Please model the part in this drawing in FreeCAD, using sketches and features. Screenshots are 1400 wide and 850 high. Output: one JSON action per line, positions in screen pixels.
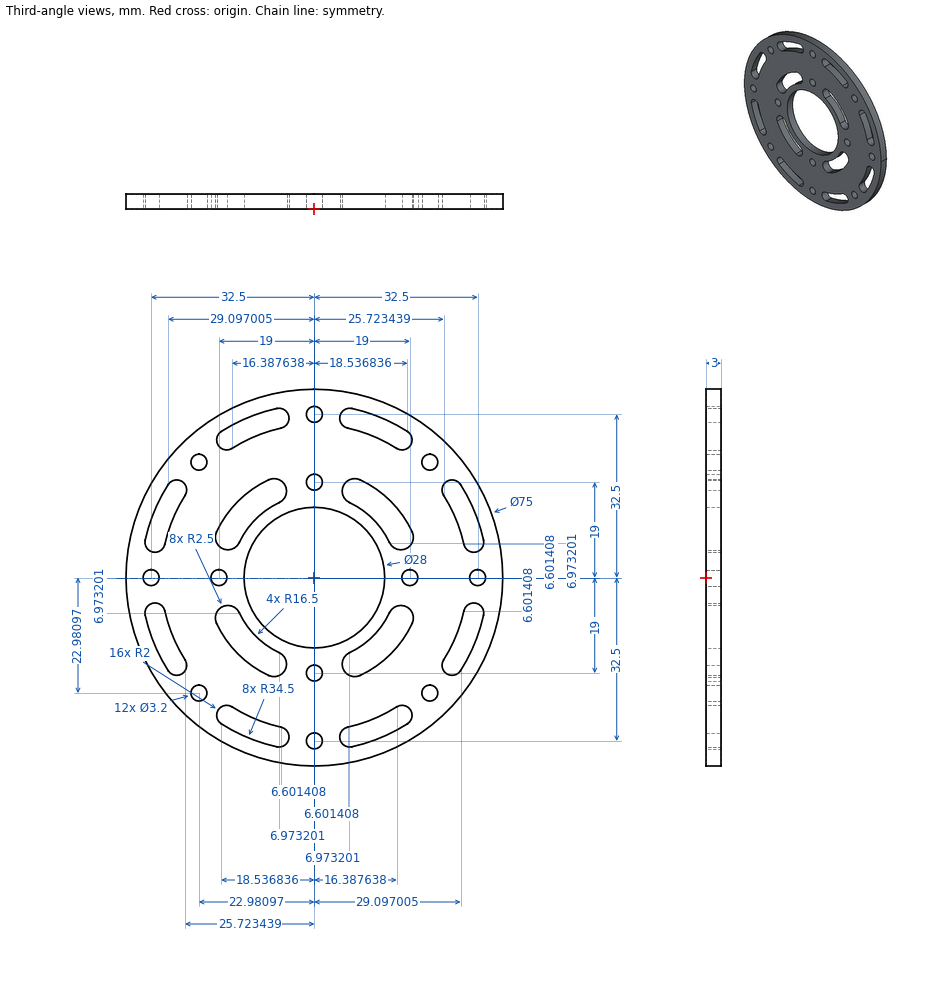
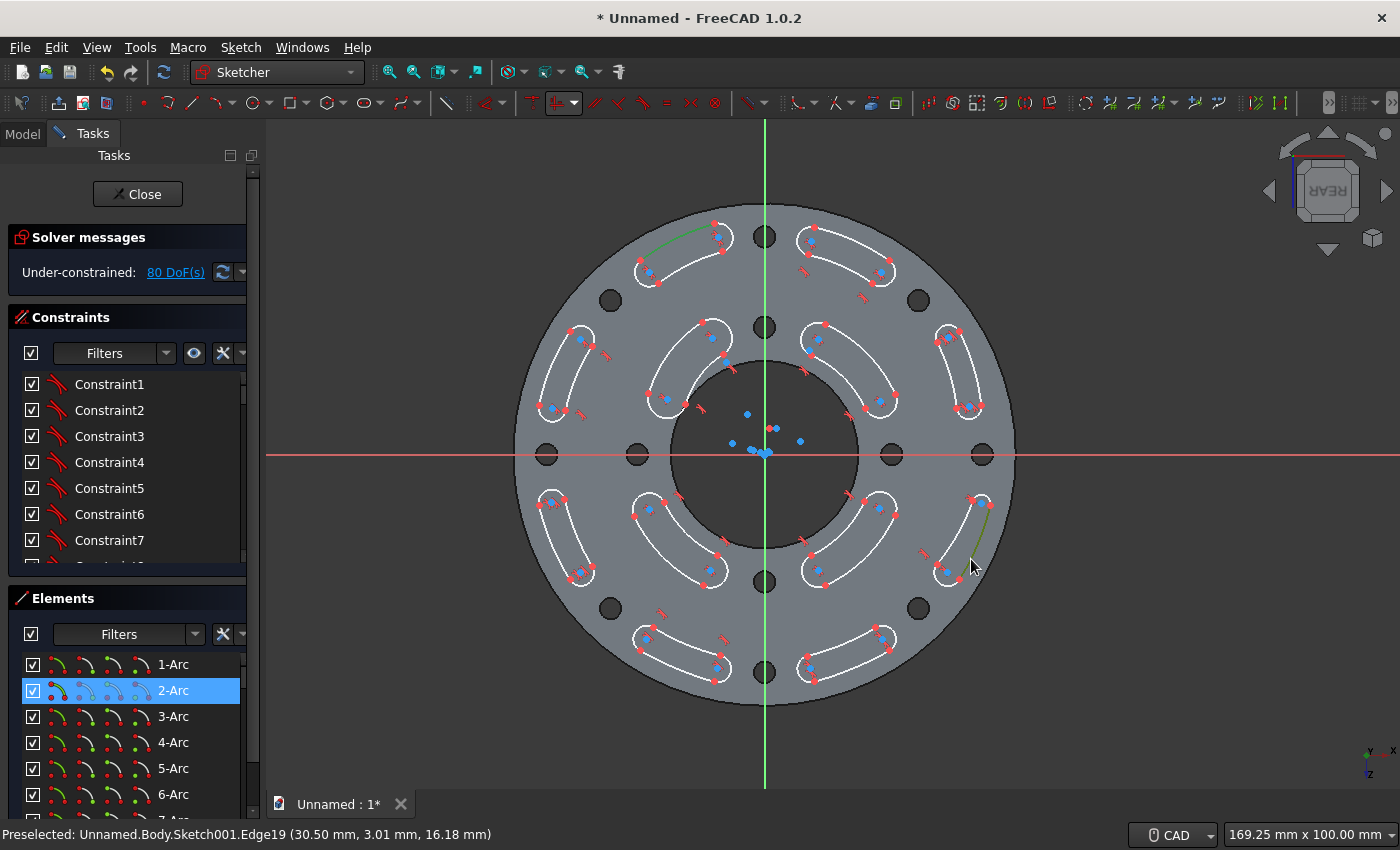
{"action": "left_click", "coordinate": [532, 104]}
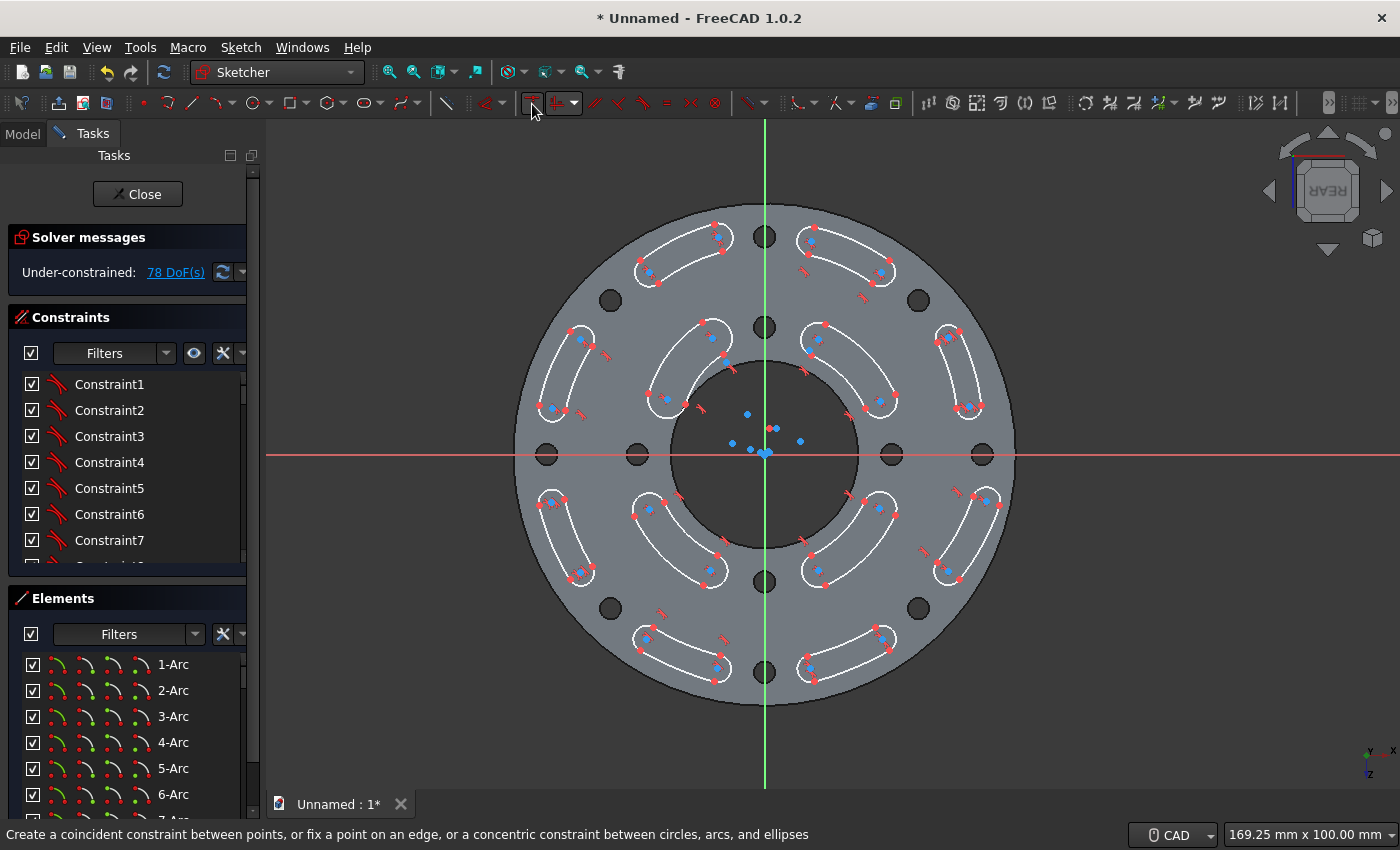
{"action": "left_click", "coordinate": [691, 232]}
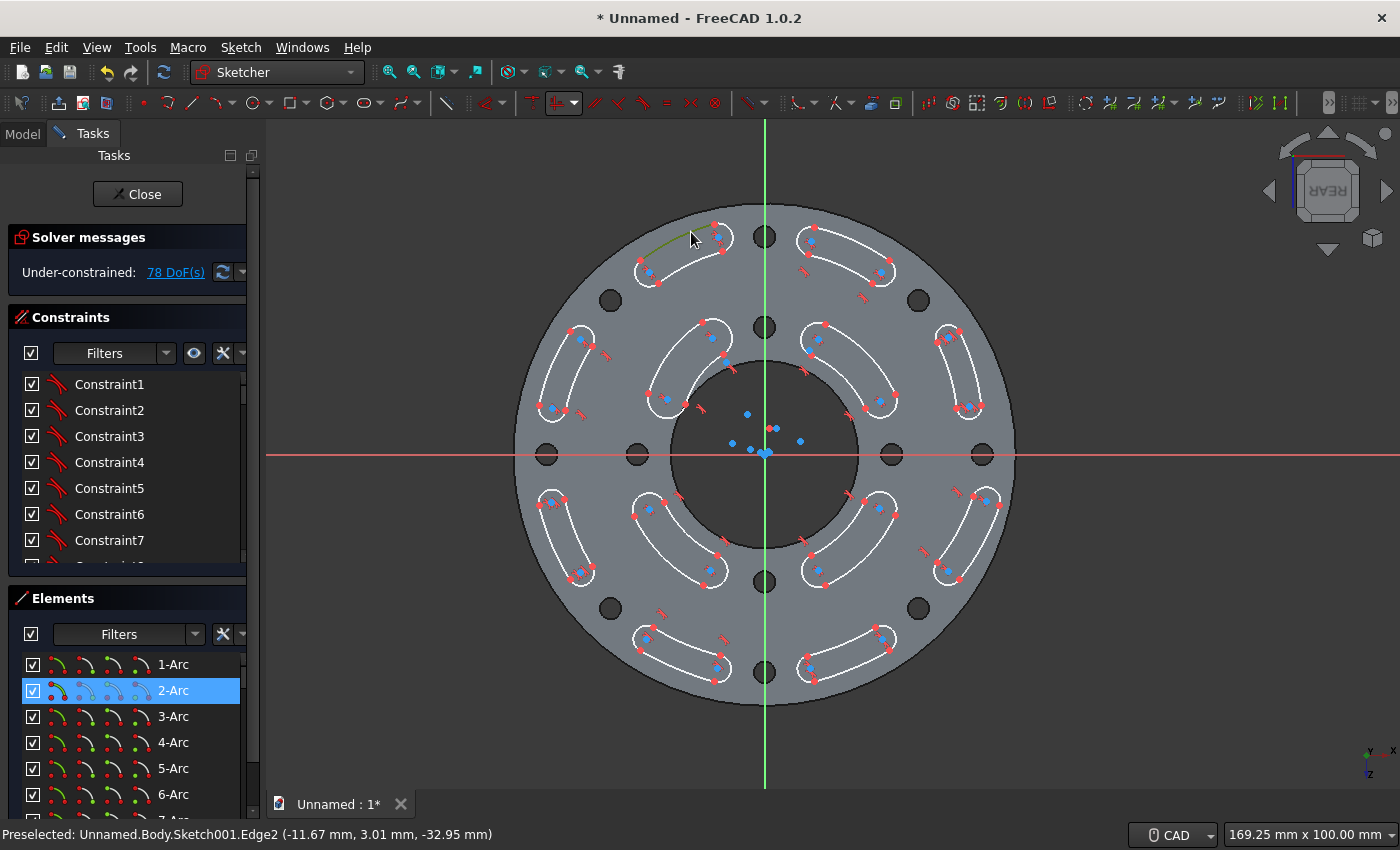
{"action": "left_click", "coordinate": [838, 674]}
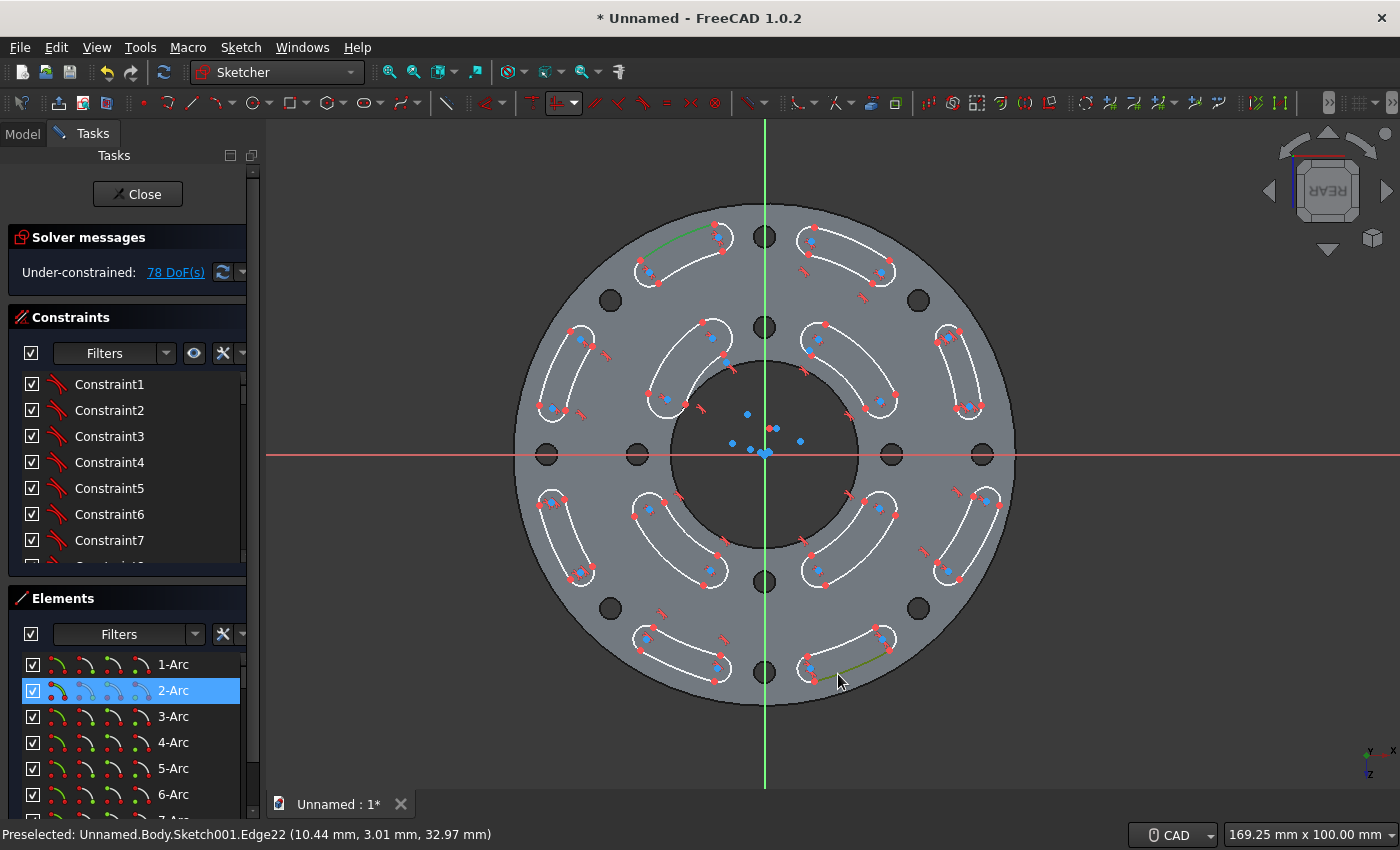
{"action": "left_click", "coordinate": [532, 104]}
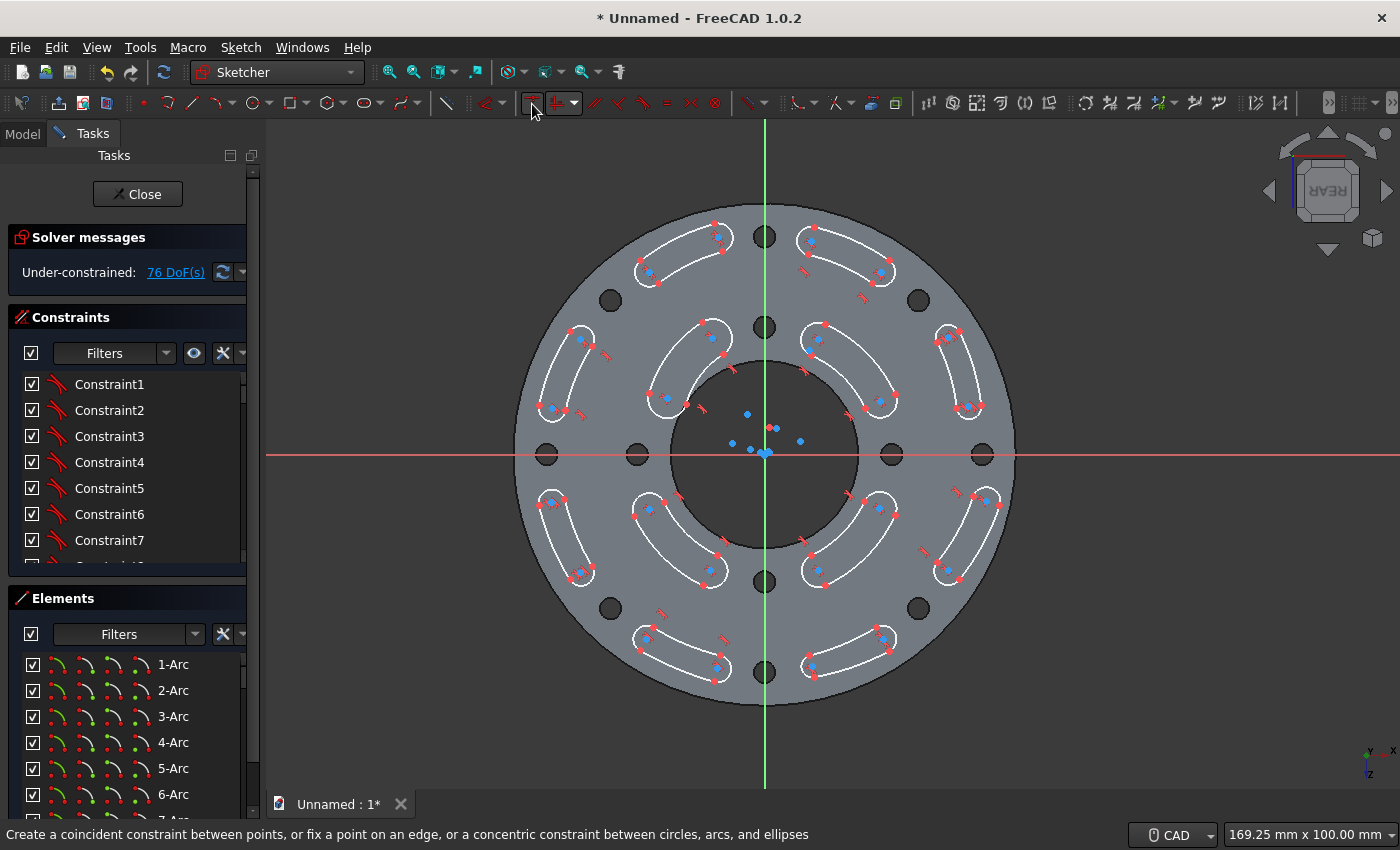
{"action": "left_click", "coordinate": [691, 232]}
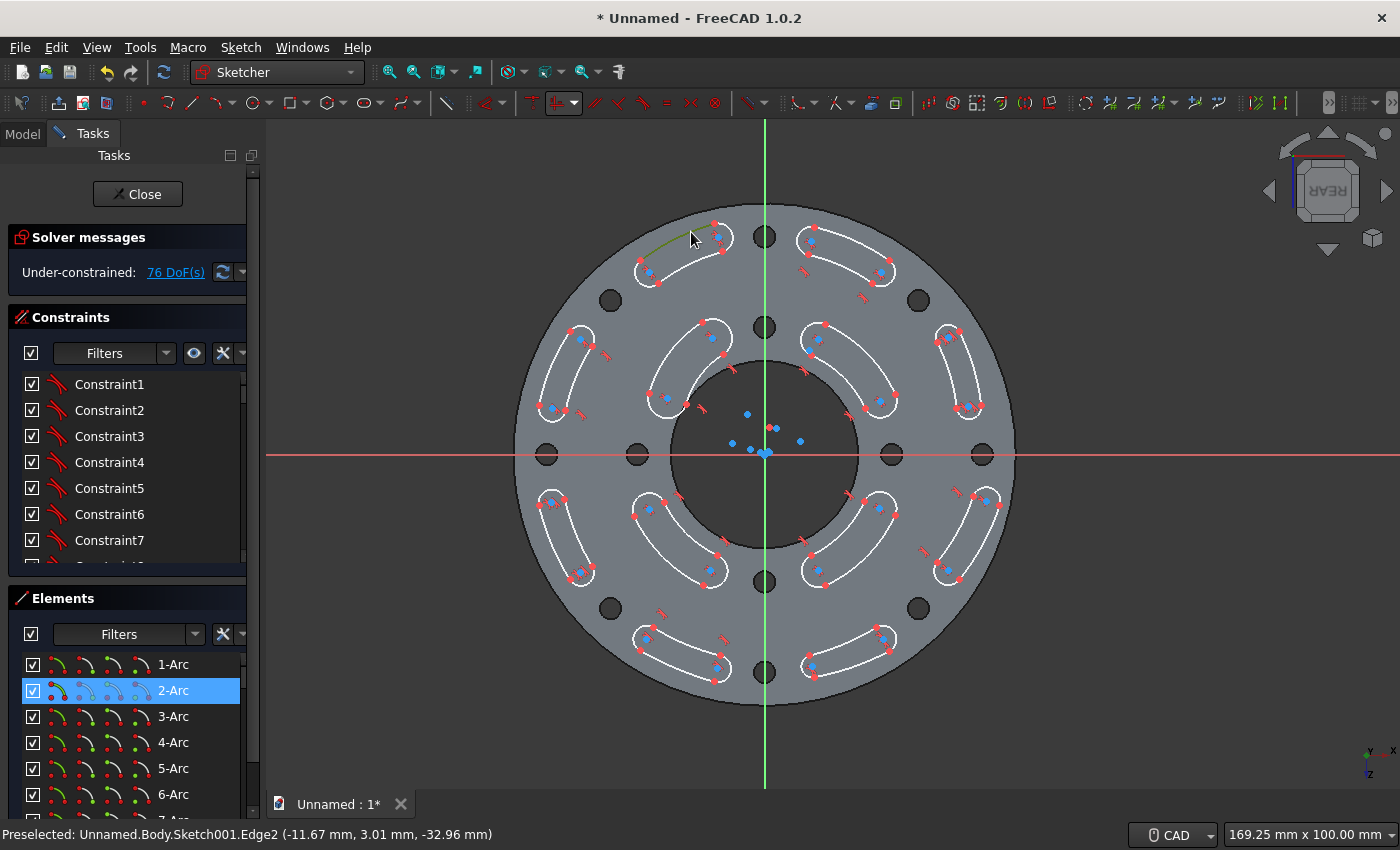
{"action": "left_click", "coordinate": [830, 649]}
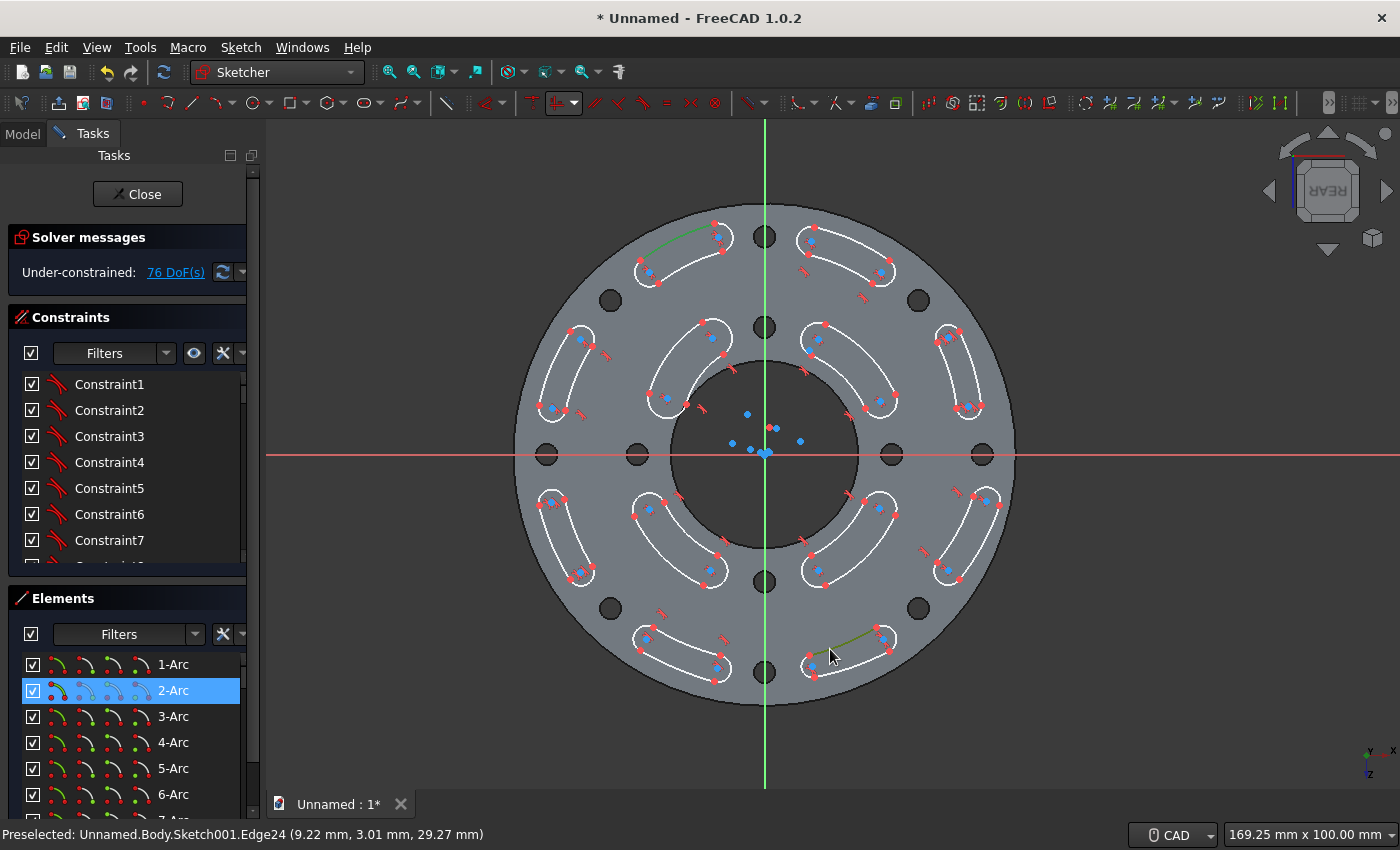
{"action": "left_click", "coordinate": [532, 104]}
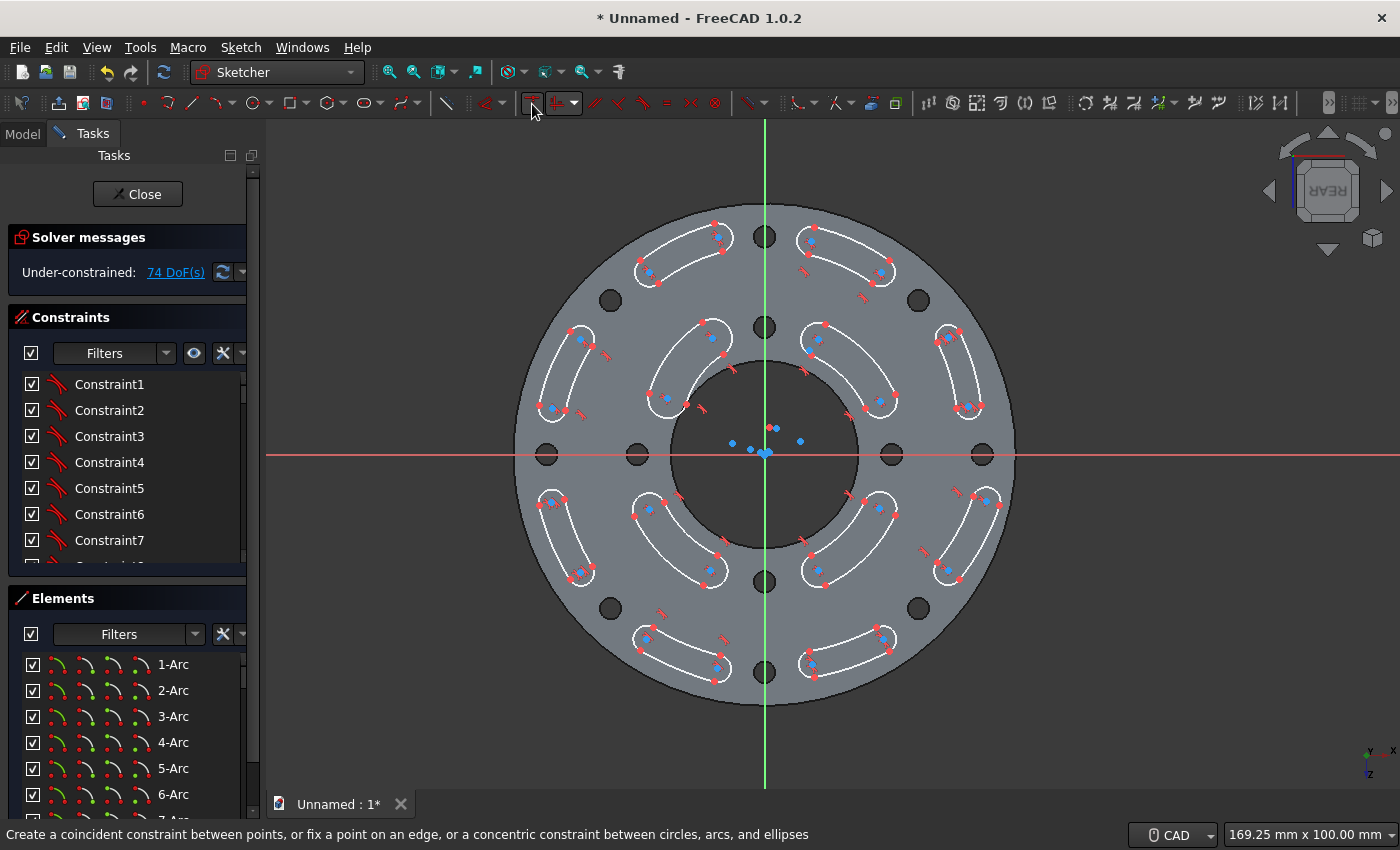
{"action": "left_click", "coordinate": [691, 232]}